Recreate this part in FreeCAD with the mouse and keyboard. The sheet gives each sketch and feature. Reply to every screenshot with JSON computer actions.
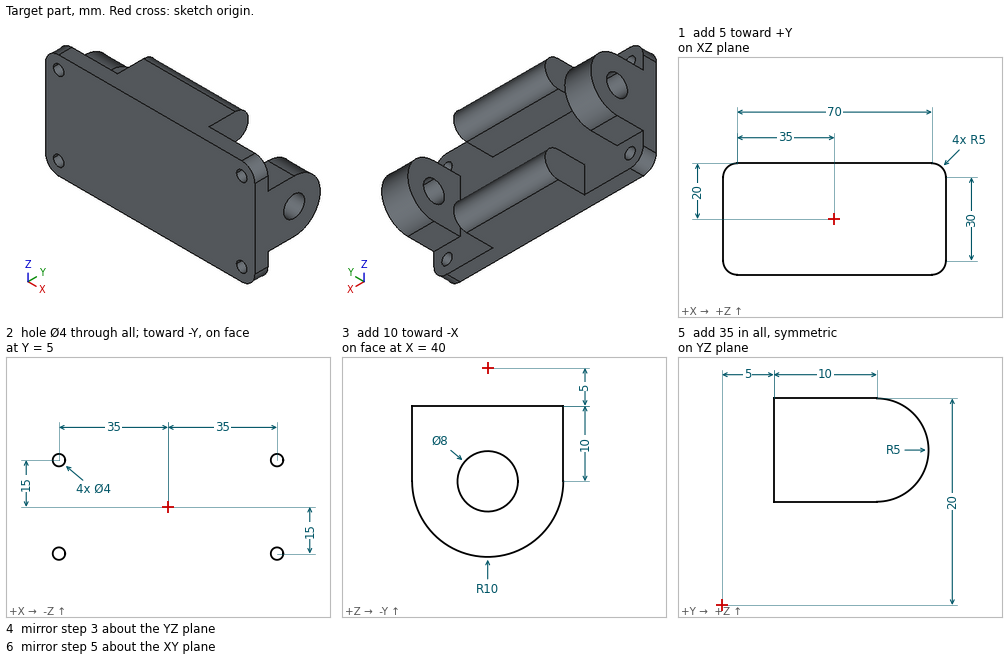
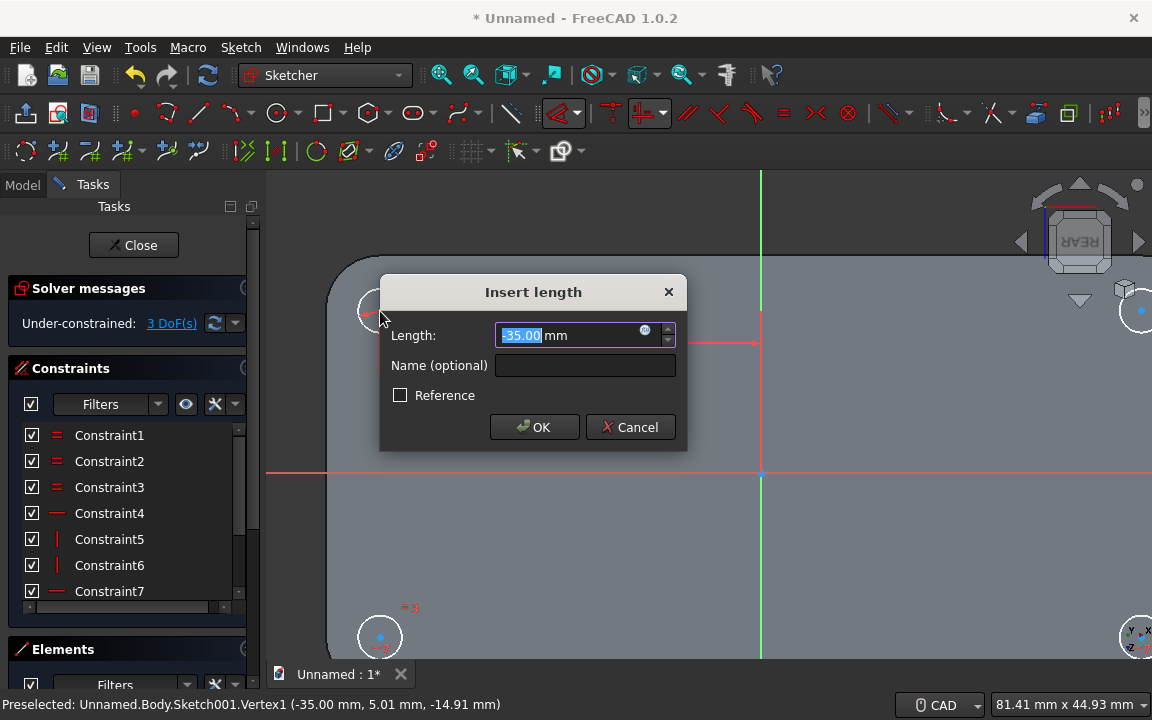
{"action": "type", "text": "-35"}
{"action": "key", "text": "Return"}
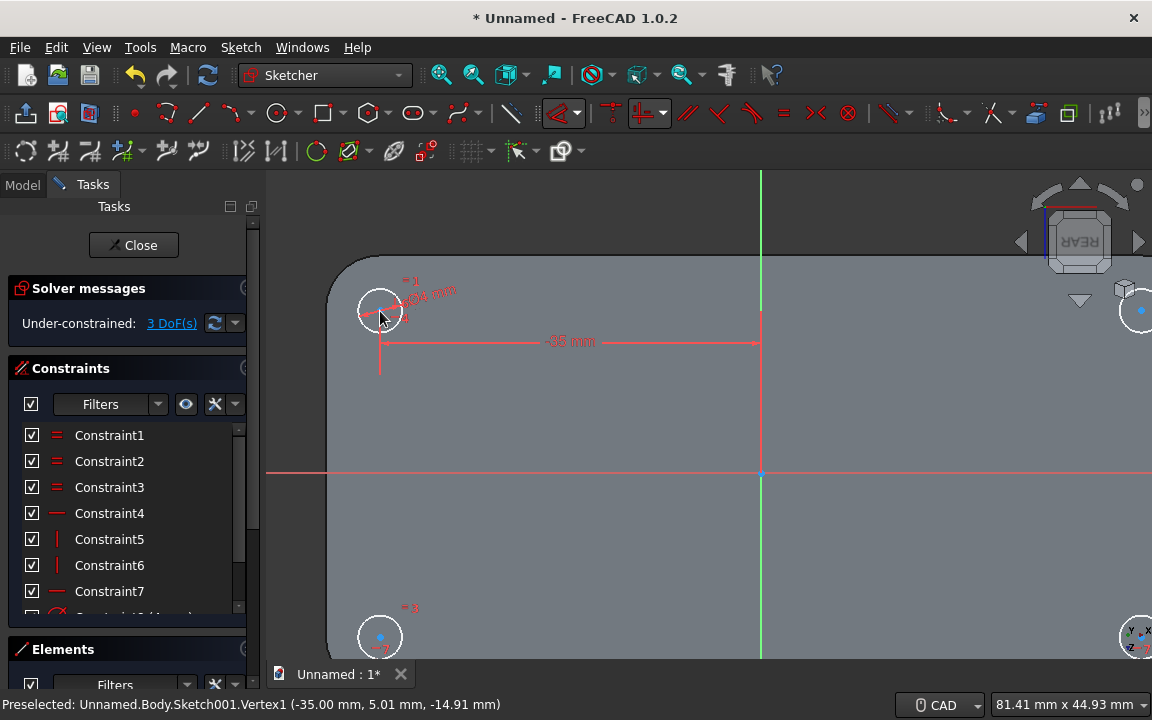
{"action": "left_click", "coordinate": [380, 311]}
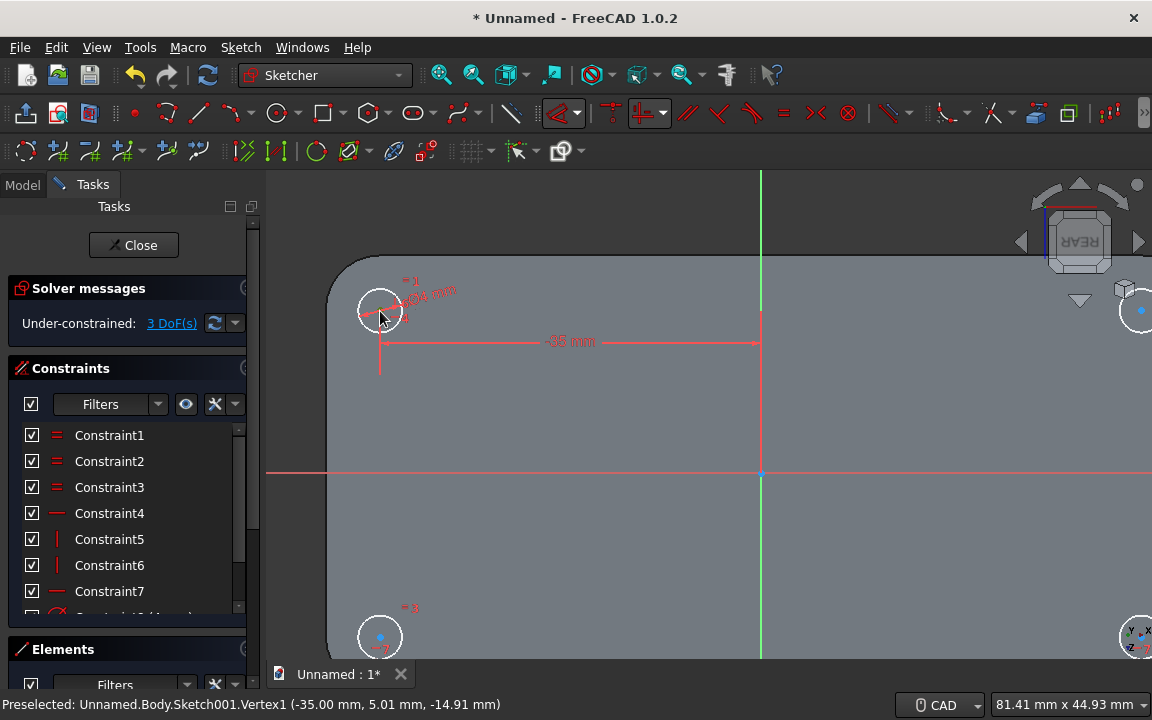
{"action": "key", "text": "i"}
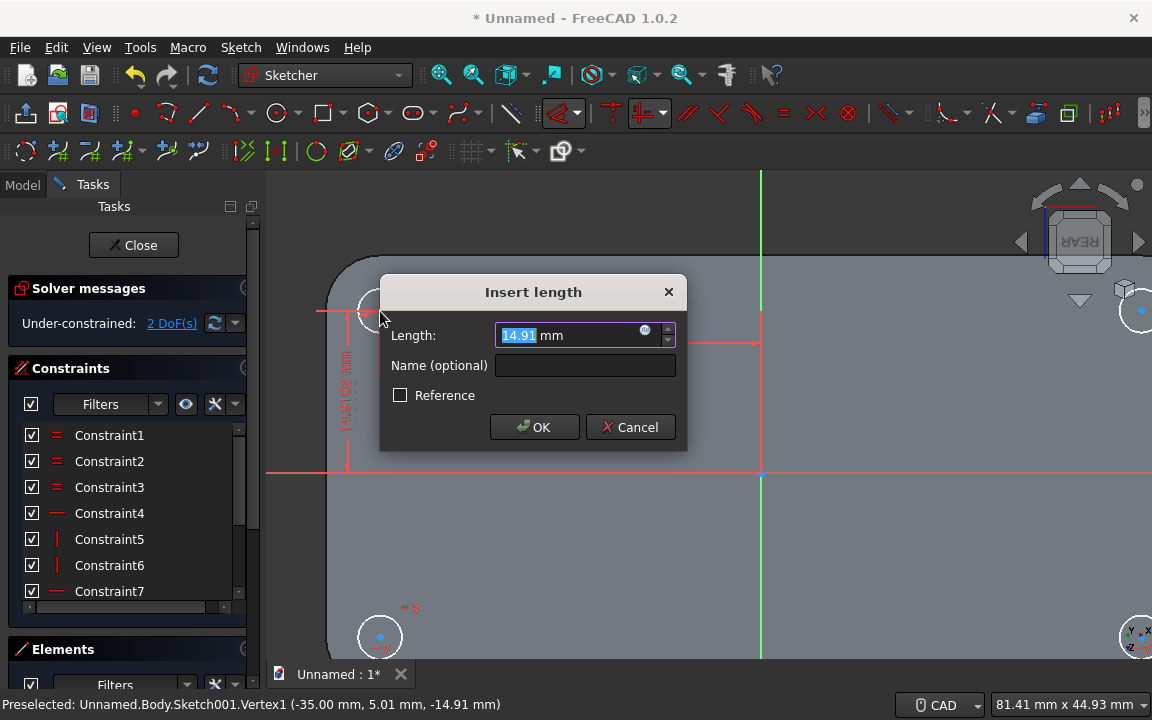
{"action": "type", "text": "15"}
{"action": "key", "text": "Return"}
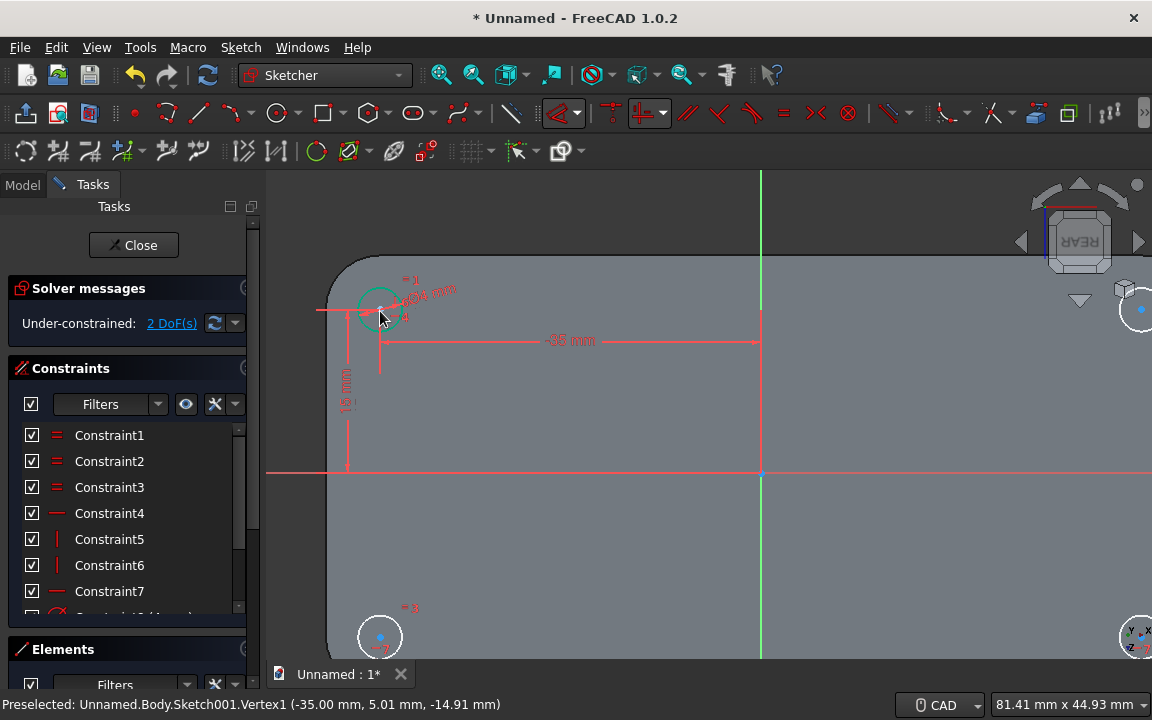
{"action": "scroll", "coordinate": [395, 295], "scroll_direction": "down", "scroll_amount": 2}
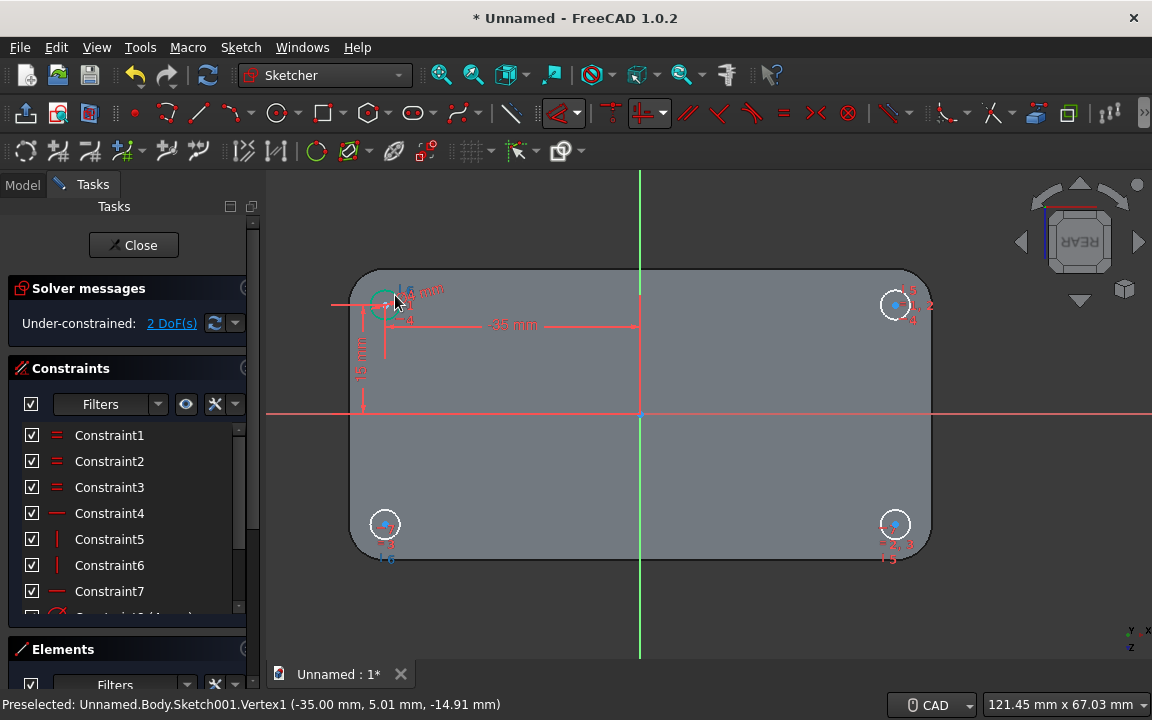
{"action": "left_click", "coordinate": [895, 305]}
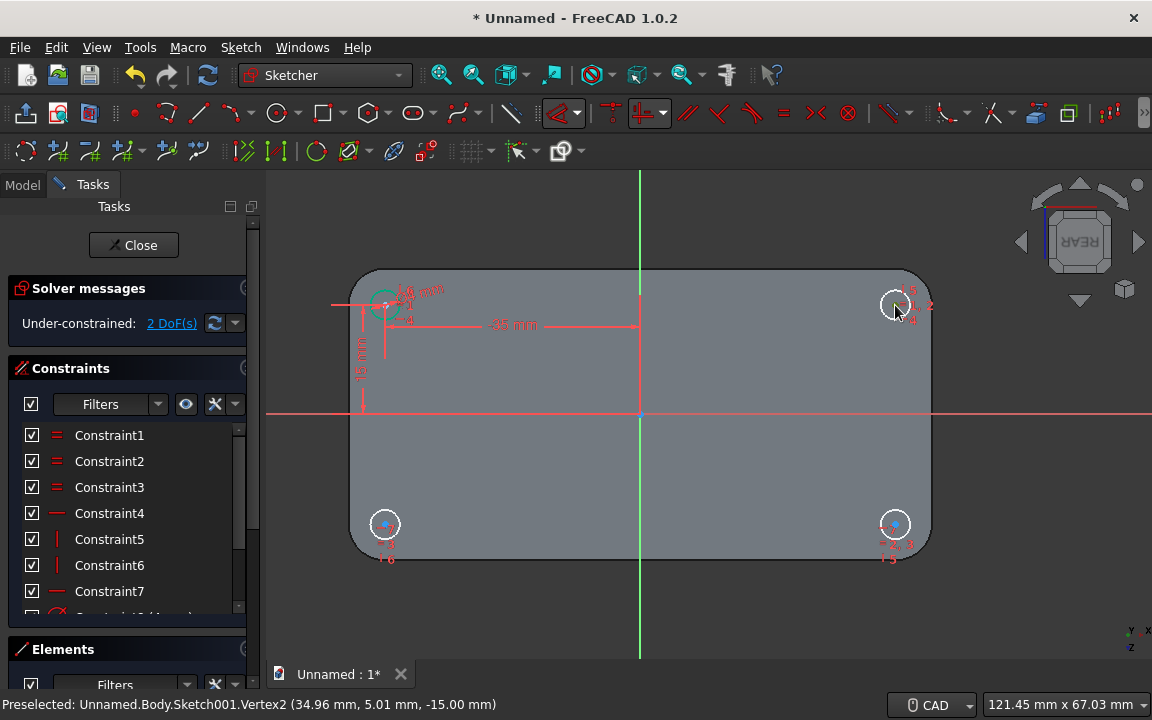
{"action": "left_click", "coordinate": [580, 114]}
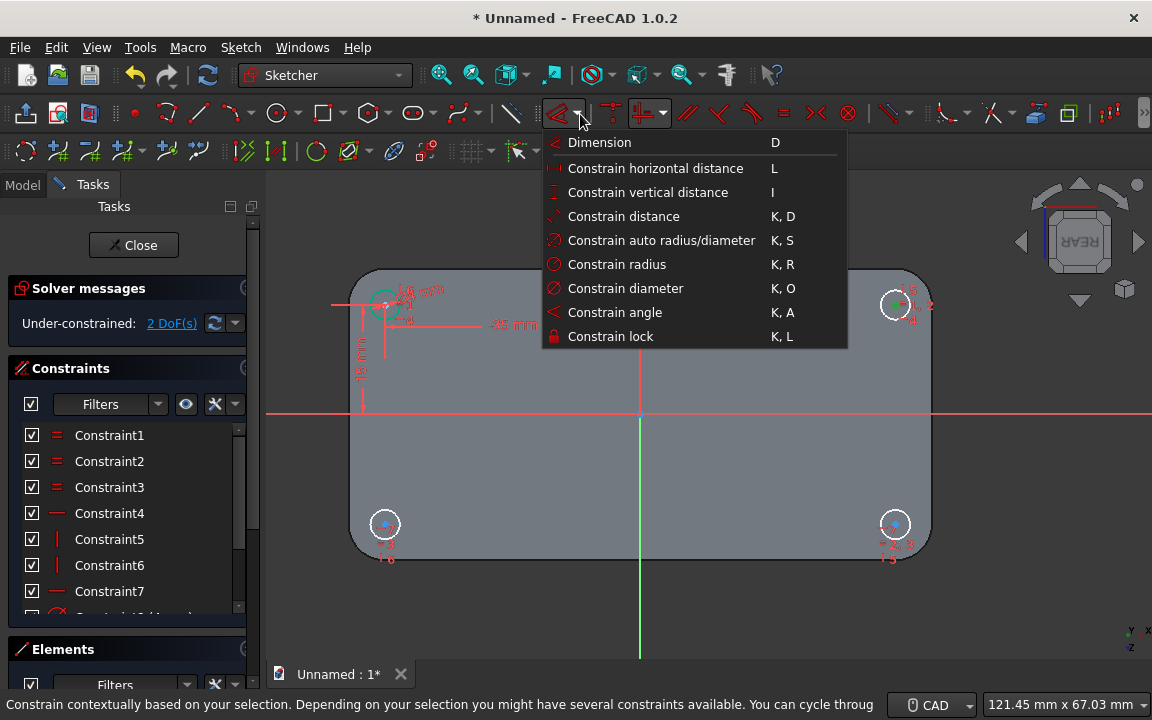
{"action": "left_click", "coordinate": [695, 168]}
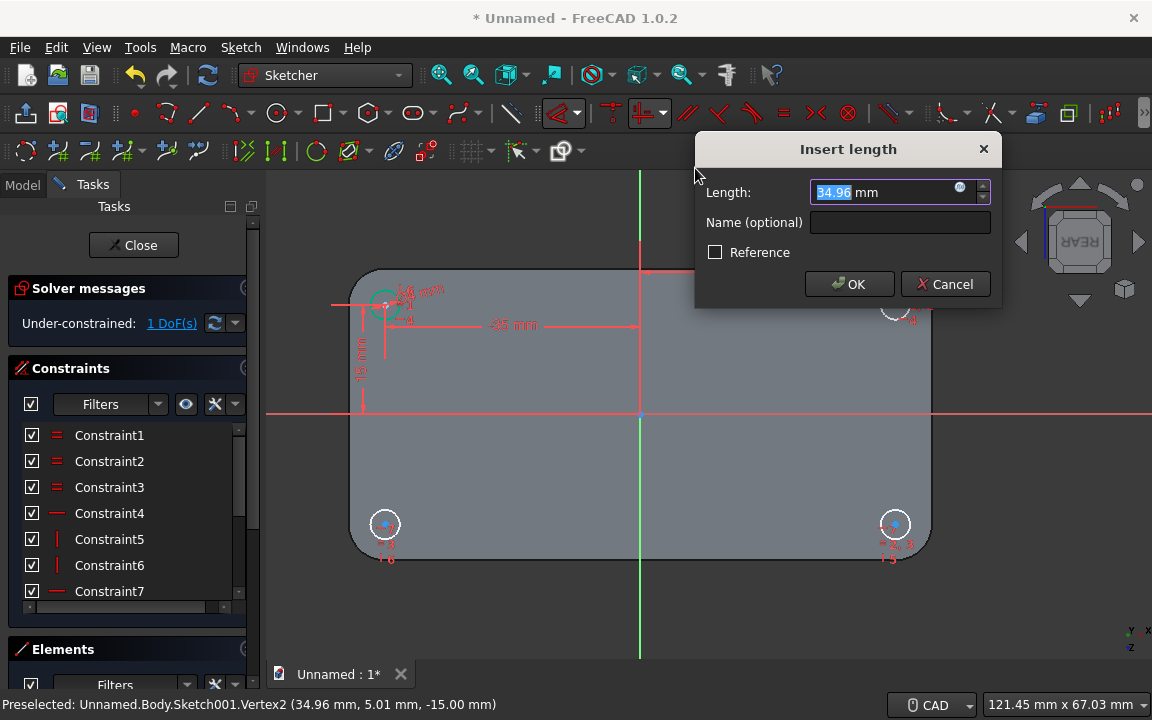
{"action": "type", "text": "35"}
{"action": "key", "text": "Return"}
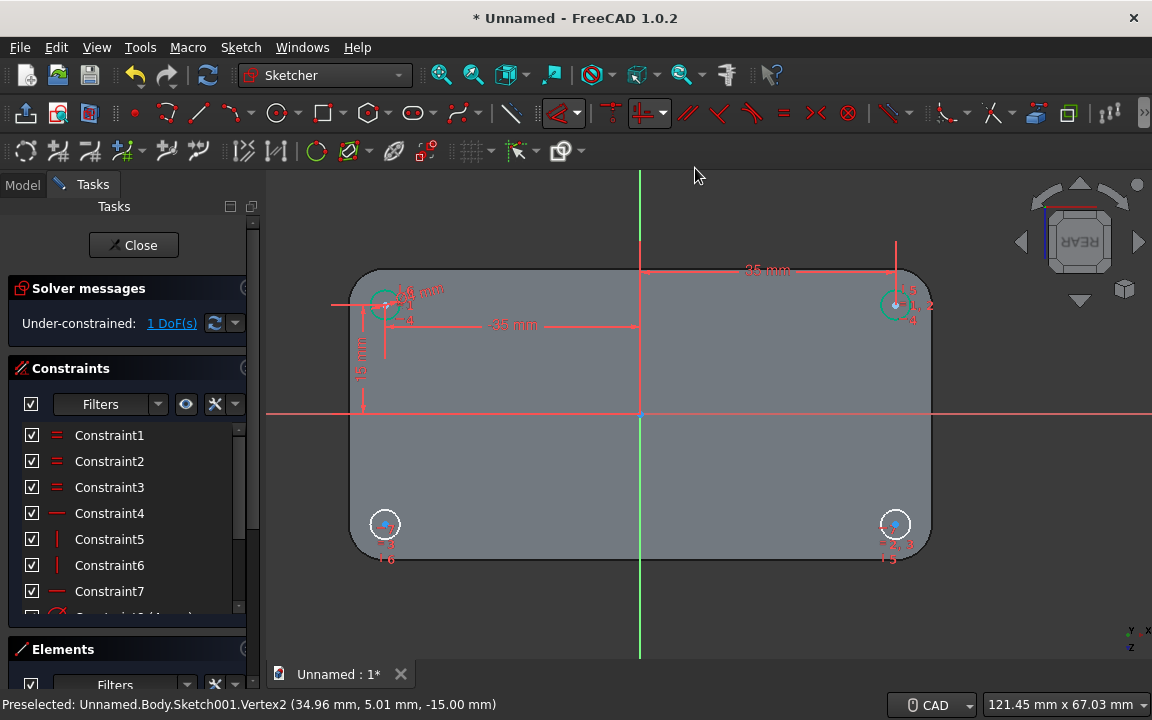
{"action": "left_click", "coordinate": [896, 525]}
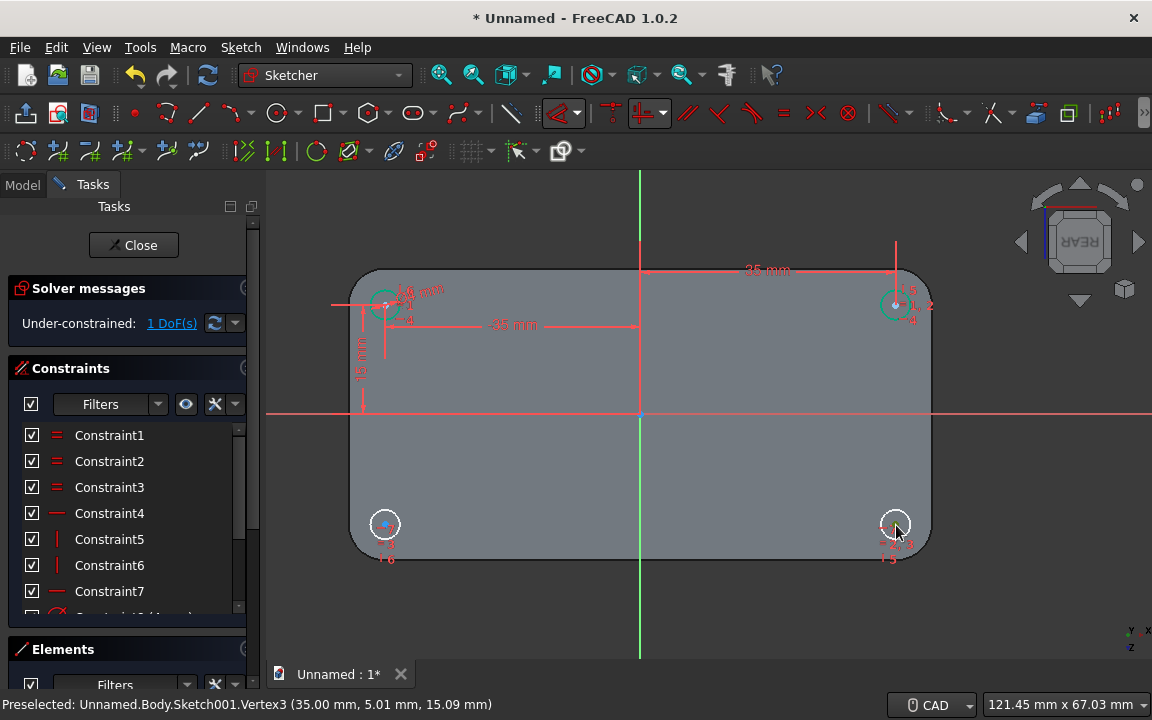
{"action": "left_click", "coordinate": [580, 114]}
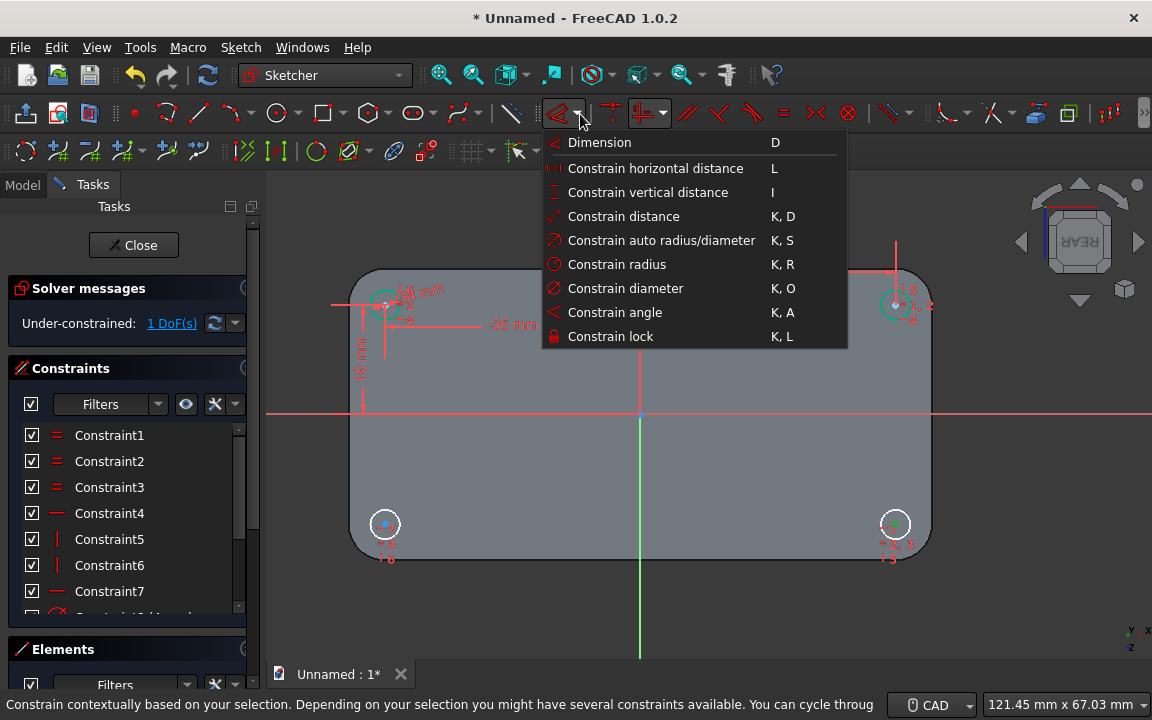
{"action": "left_click", "coordinate": [695, 192]}